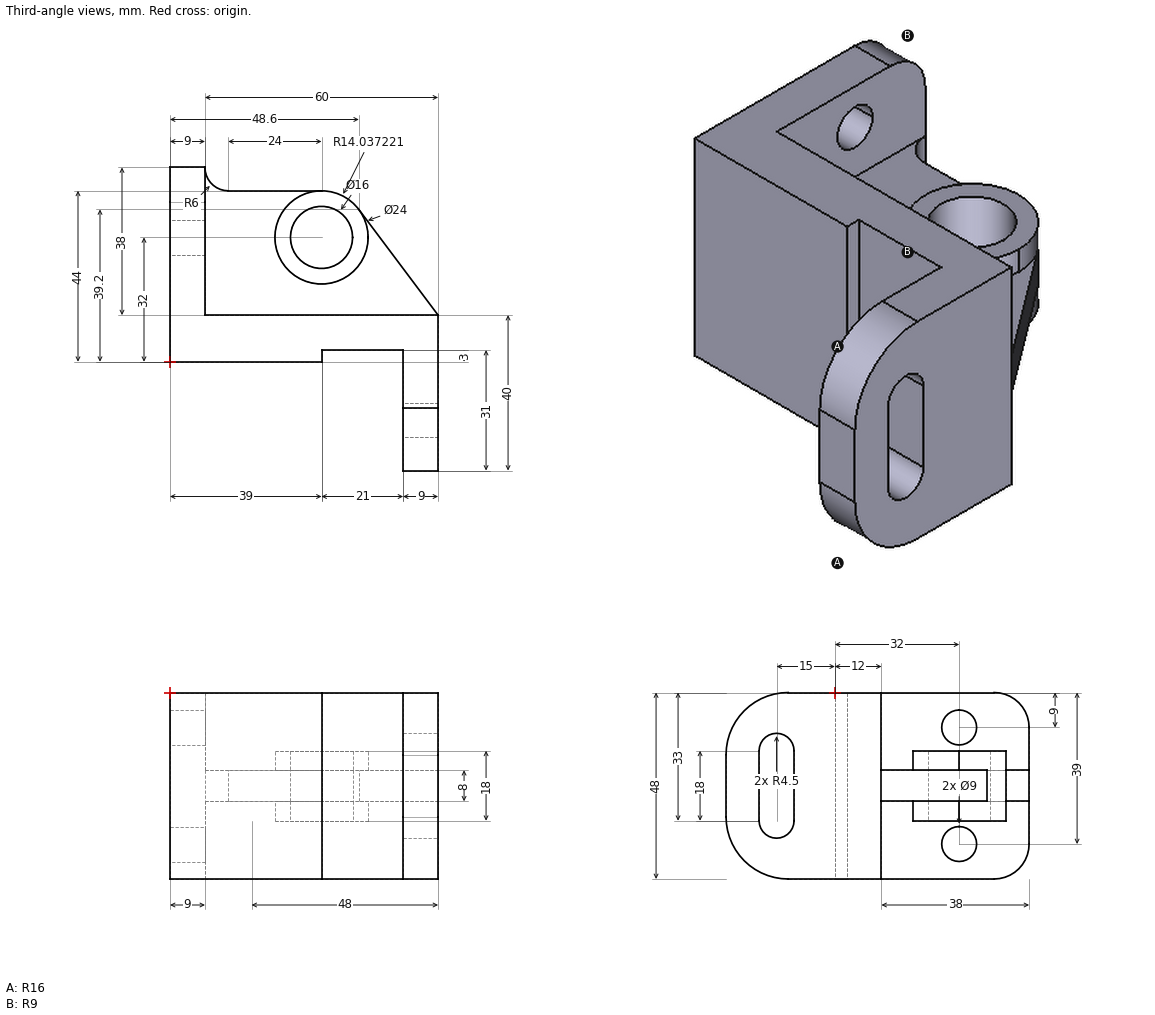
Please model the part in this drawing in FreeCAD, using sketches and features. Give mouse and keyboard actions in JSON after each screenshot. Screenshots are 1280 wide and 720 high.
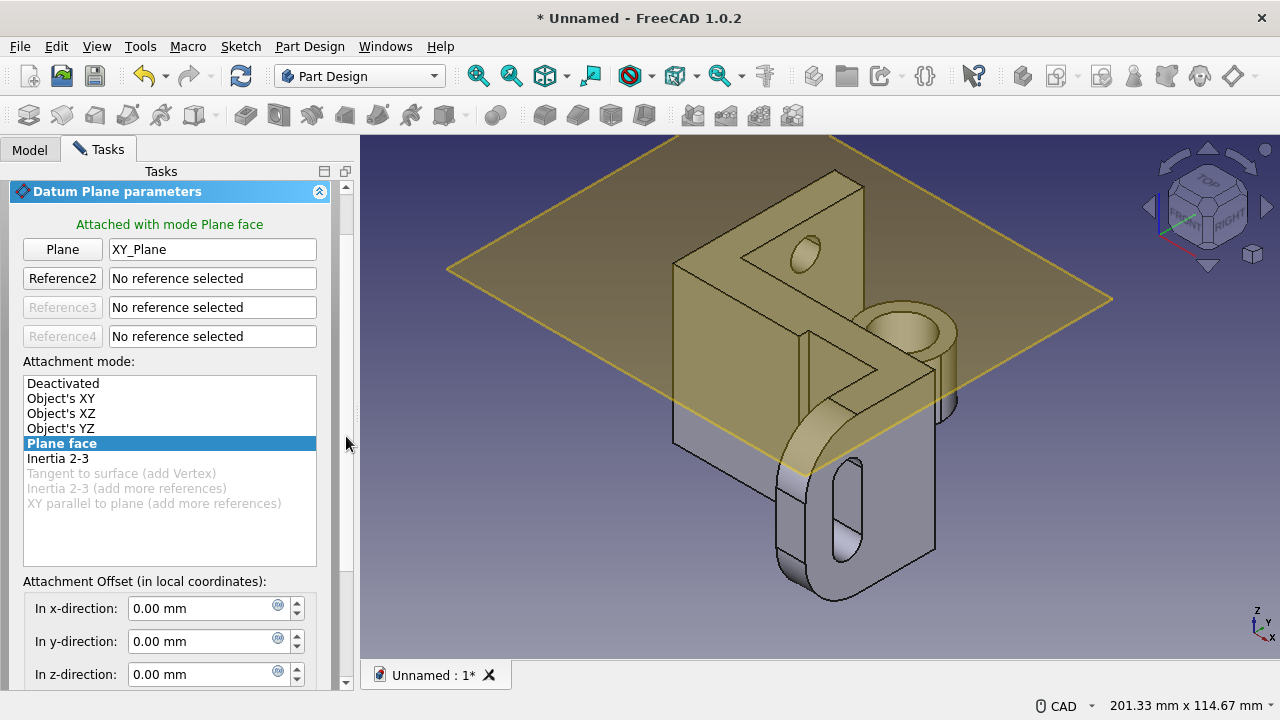
{"action": "triple_click", "coordinate": [210, 614]}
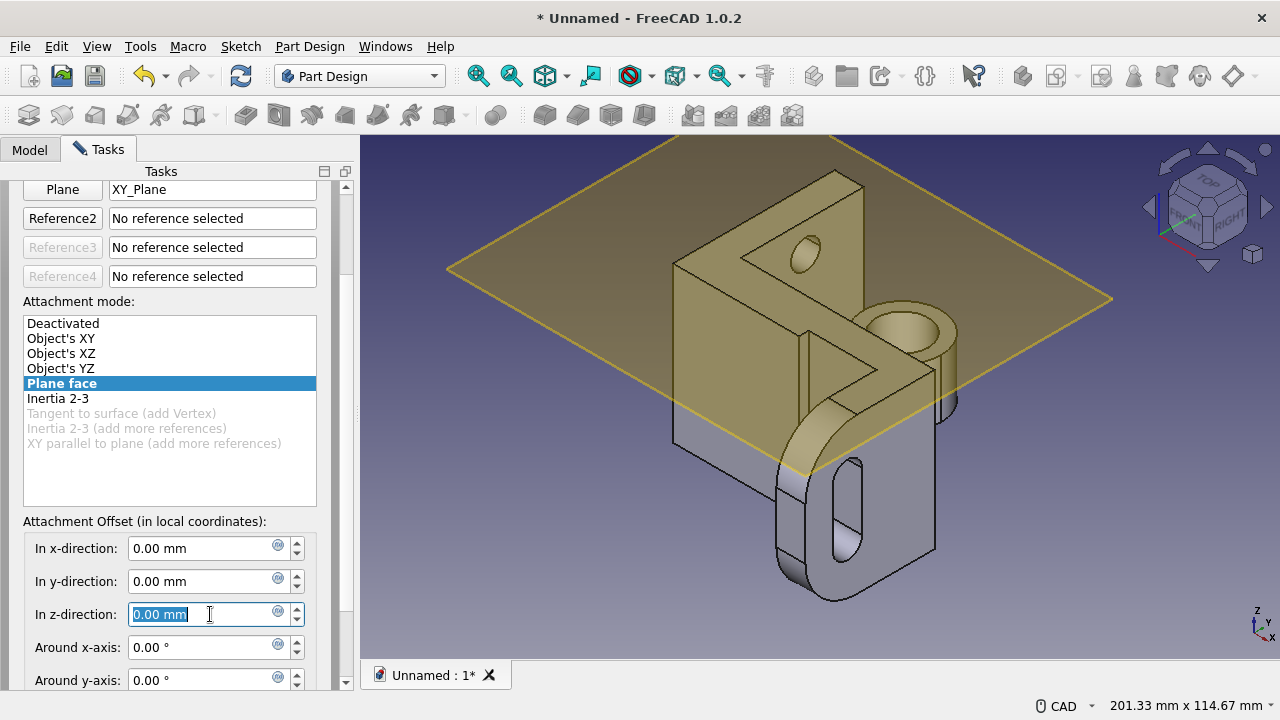
{"action": "type", "text": "-24"}
{"action": "key", "text": "Tab"}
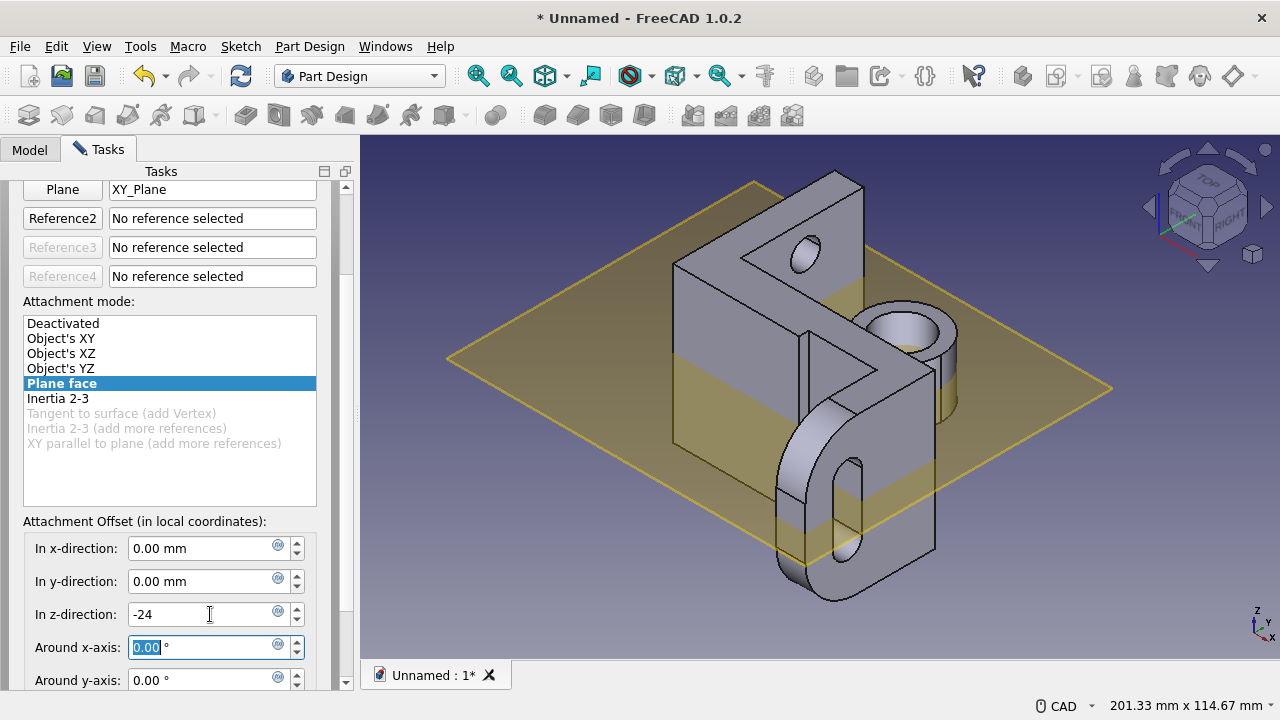
{"action": "scroll", "coordinate": [346, 436], "scroll_direction": "up", "scroll_amount": 3}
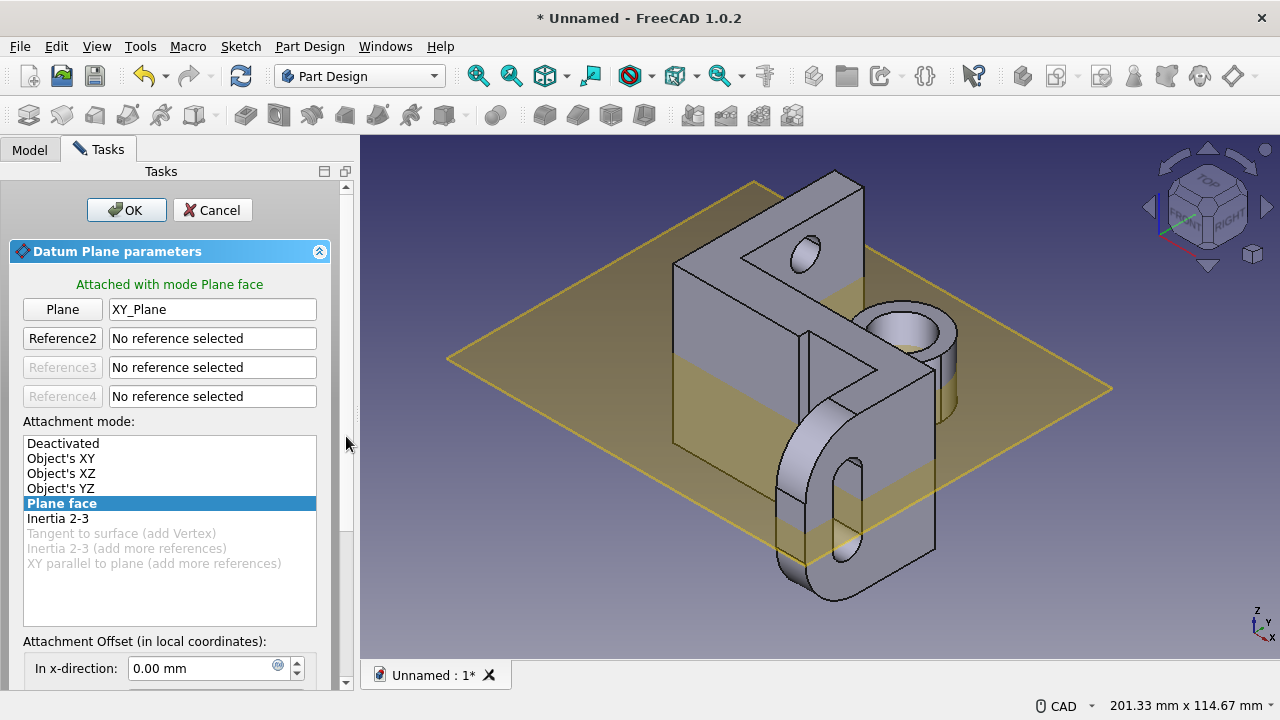
{"action": "left_click", "coordinate": [127, 210]}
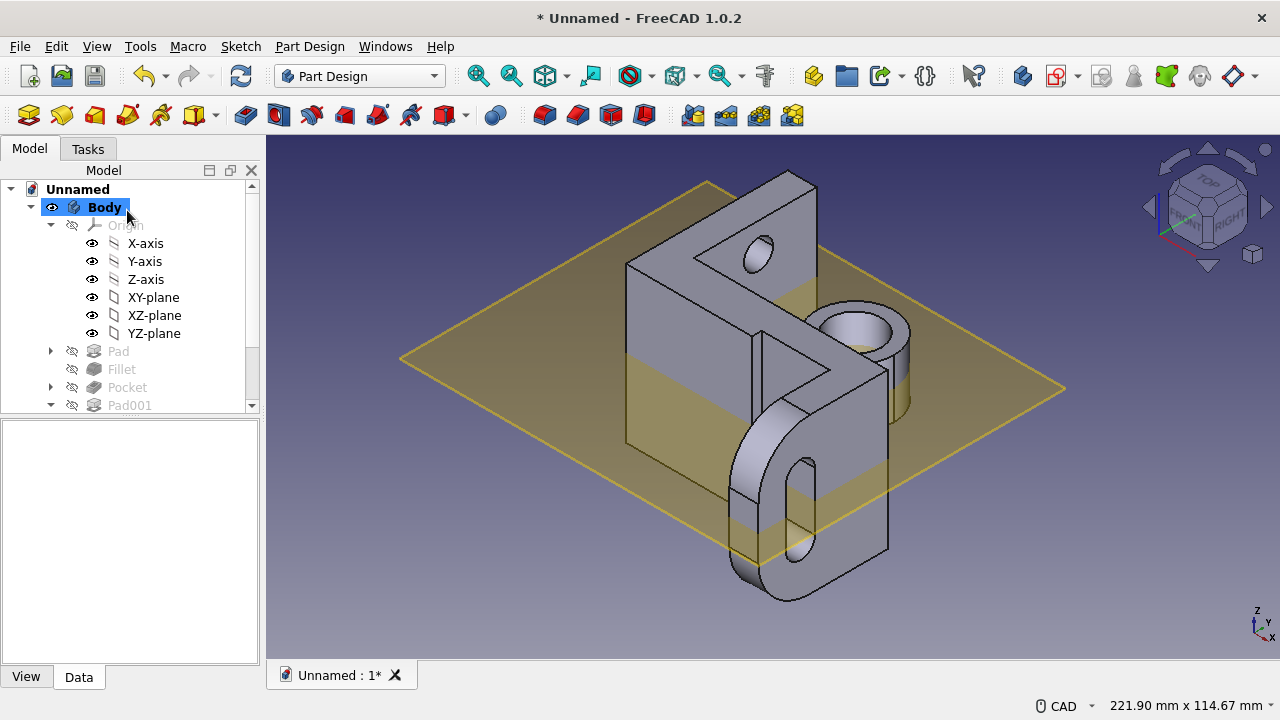
{"action": "scroll", "coordinate": [101, 293], "scroll_direction": "down", "scroll_amount": 3}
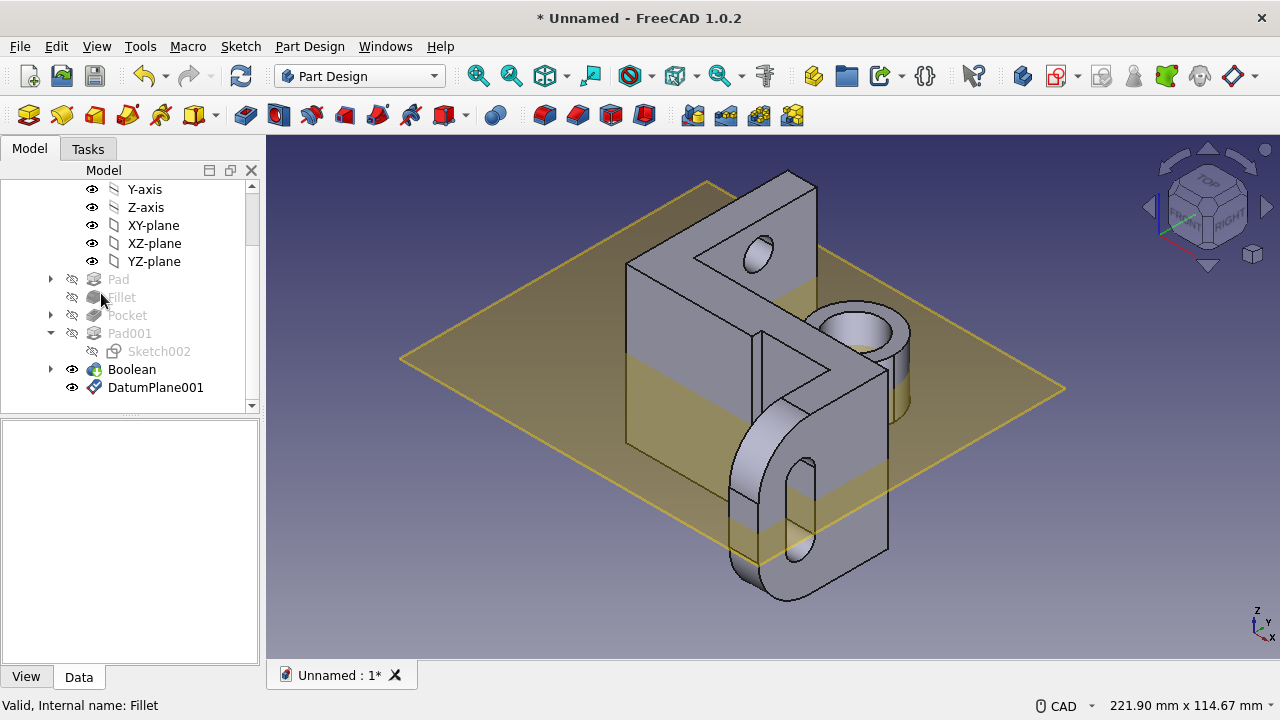
{"action": "left_click", "coordinate": [117, 387]}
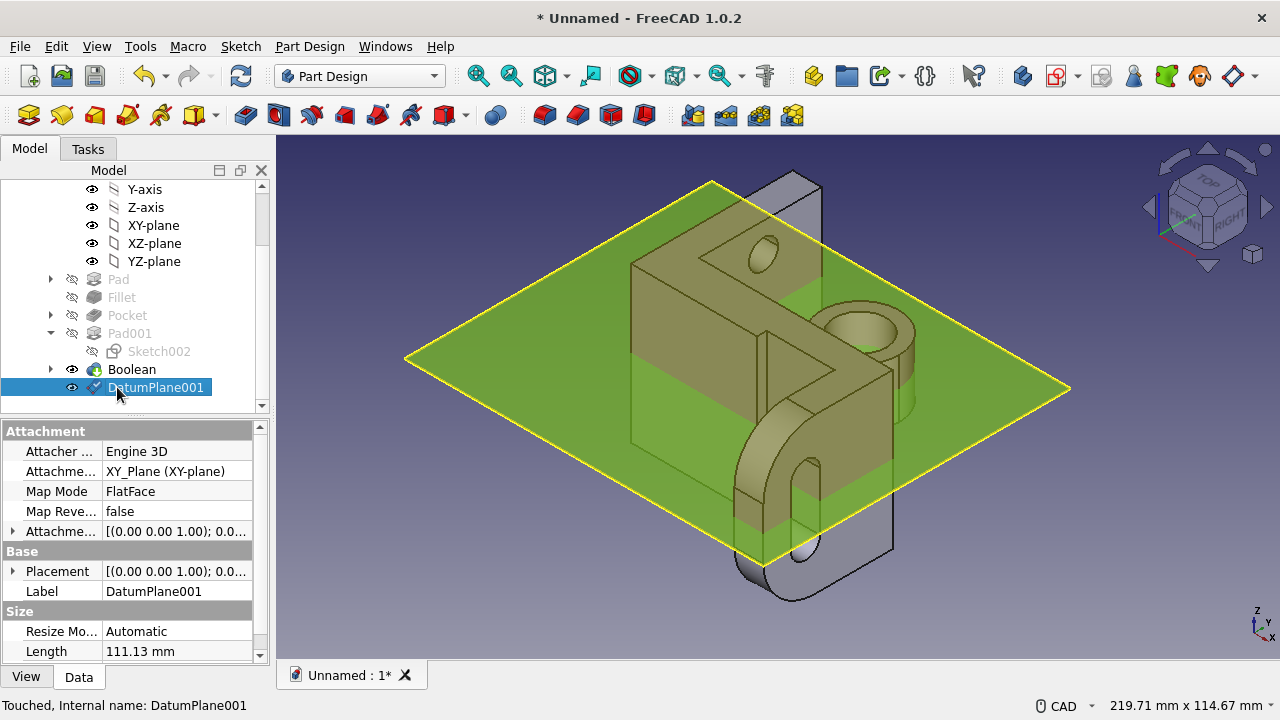
{"action": "left_click", "coordinate": [1056, 76]}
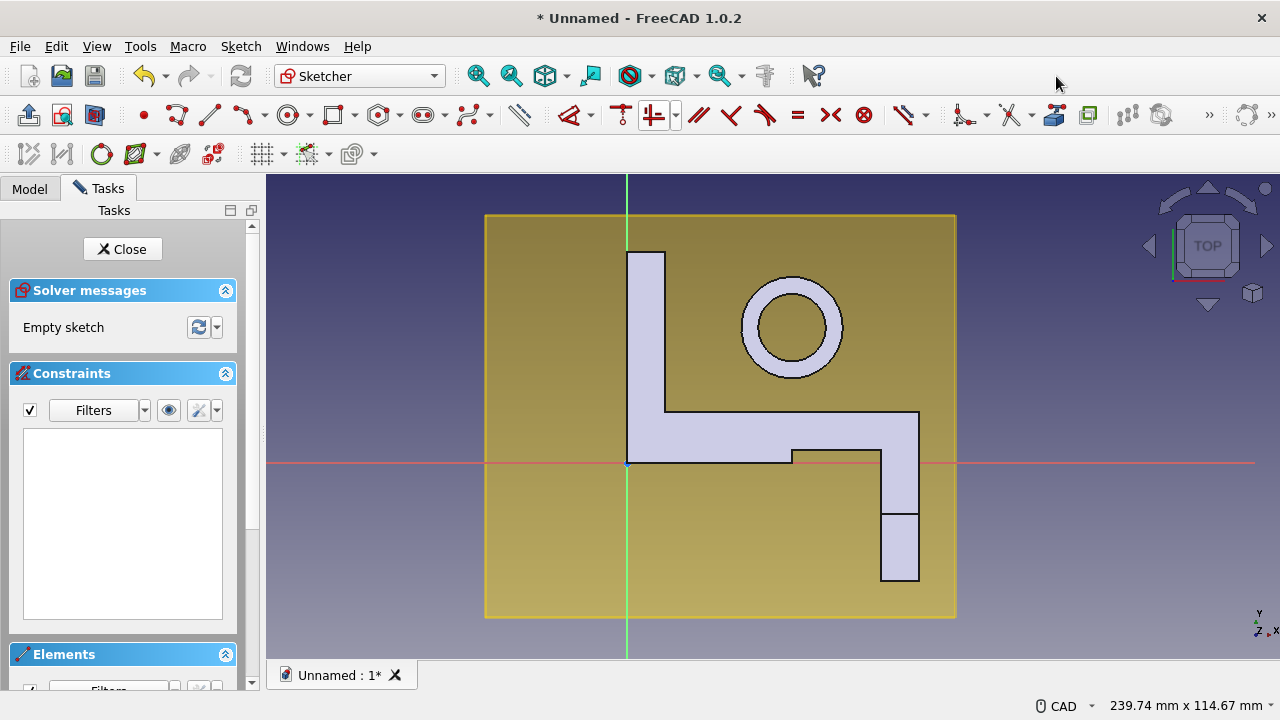
{"action": "key", "text": "q s"}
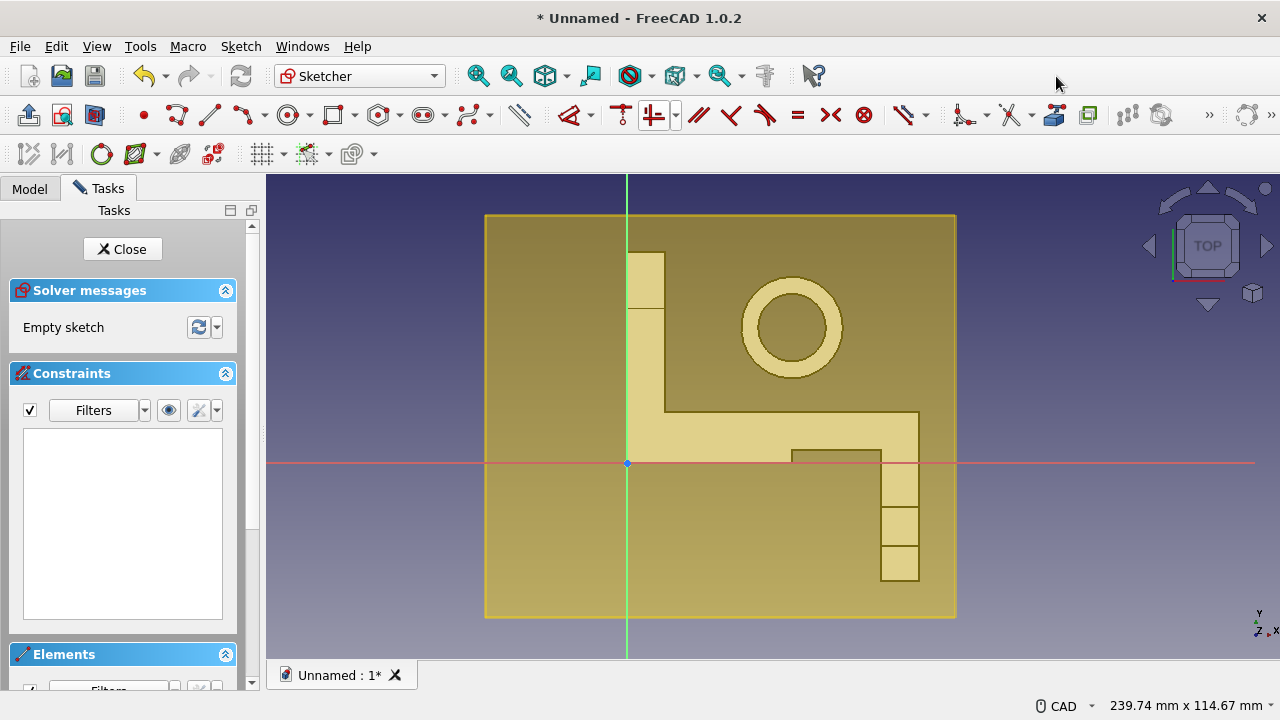
{"action": "scroll", "coordinate": [912, 237], "scroll_direction": "up", "scroll_amount": 2}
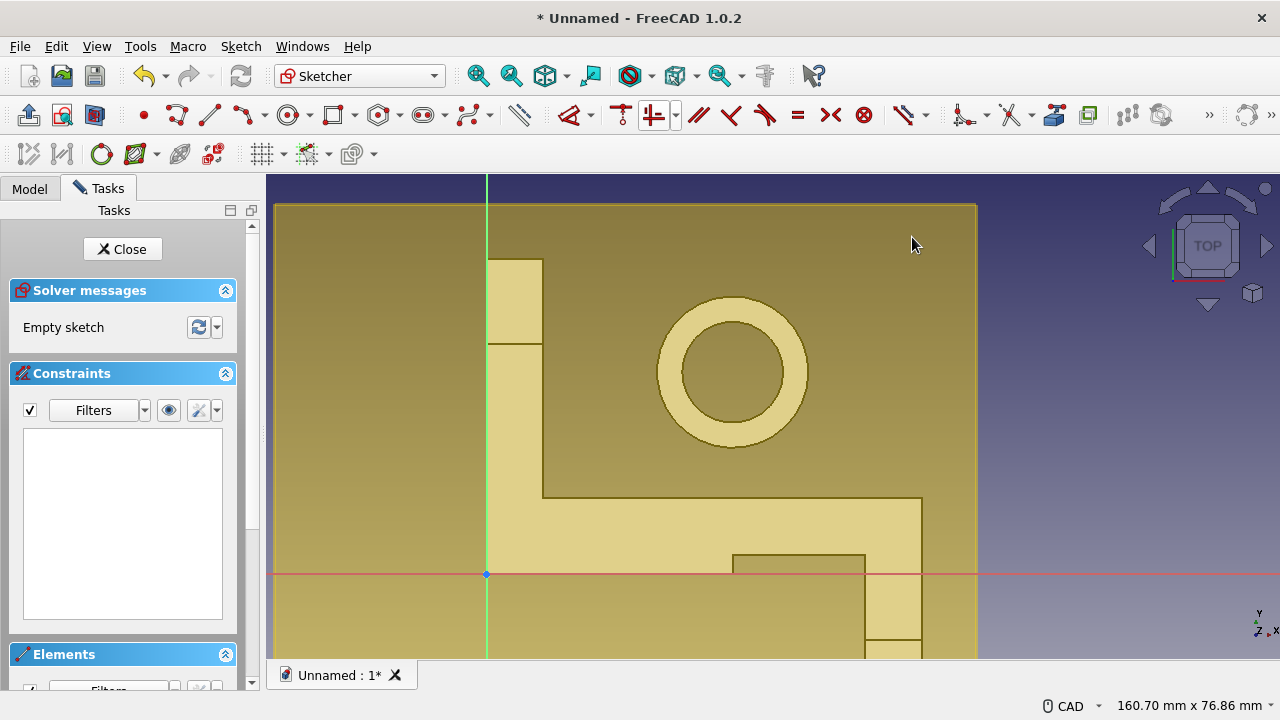
{"action": "left_click", "coordinate": [210, 116]}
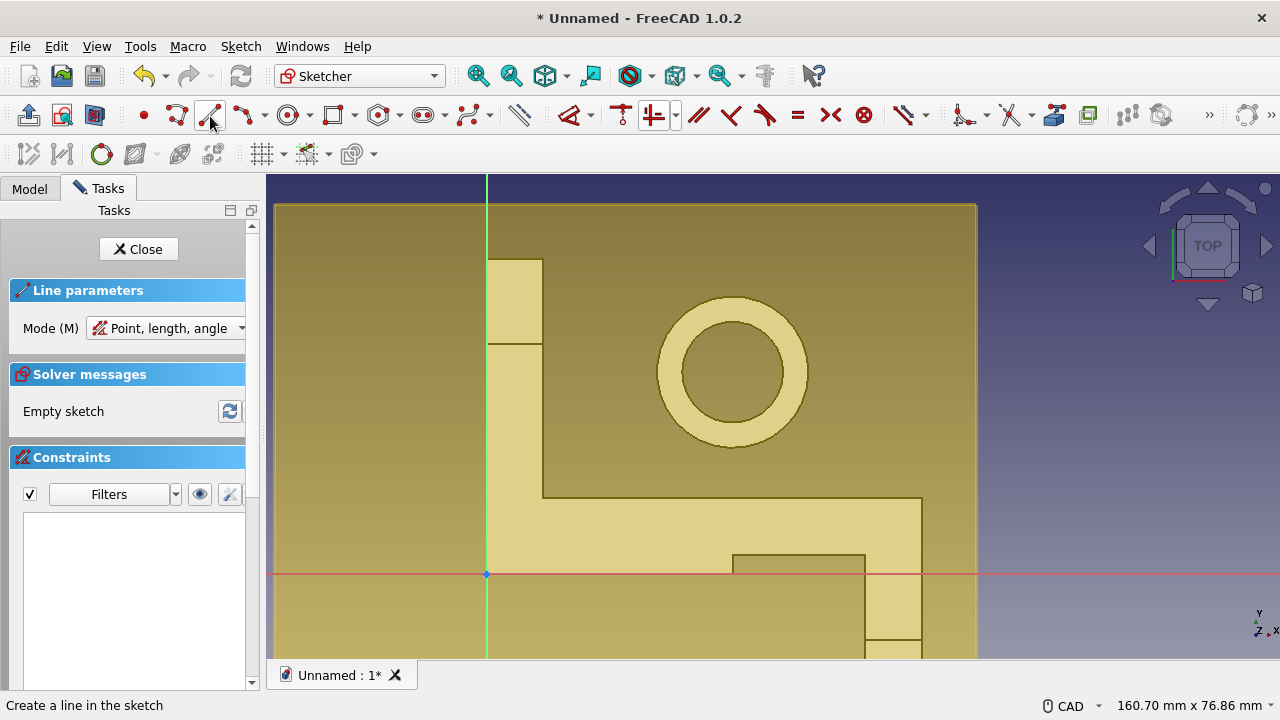
{"action": "left_click", "coordinate": [733, 296]}
{"action": "left_click", "coordinate": [581, 296]}